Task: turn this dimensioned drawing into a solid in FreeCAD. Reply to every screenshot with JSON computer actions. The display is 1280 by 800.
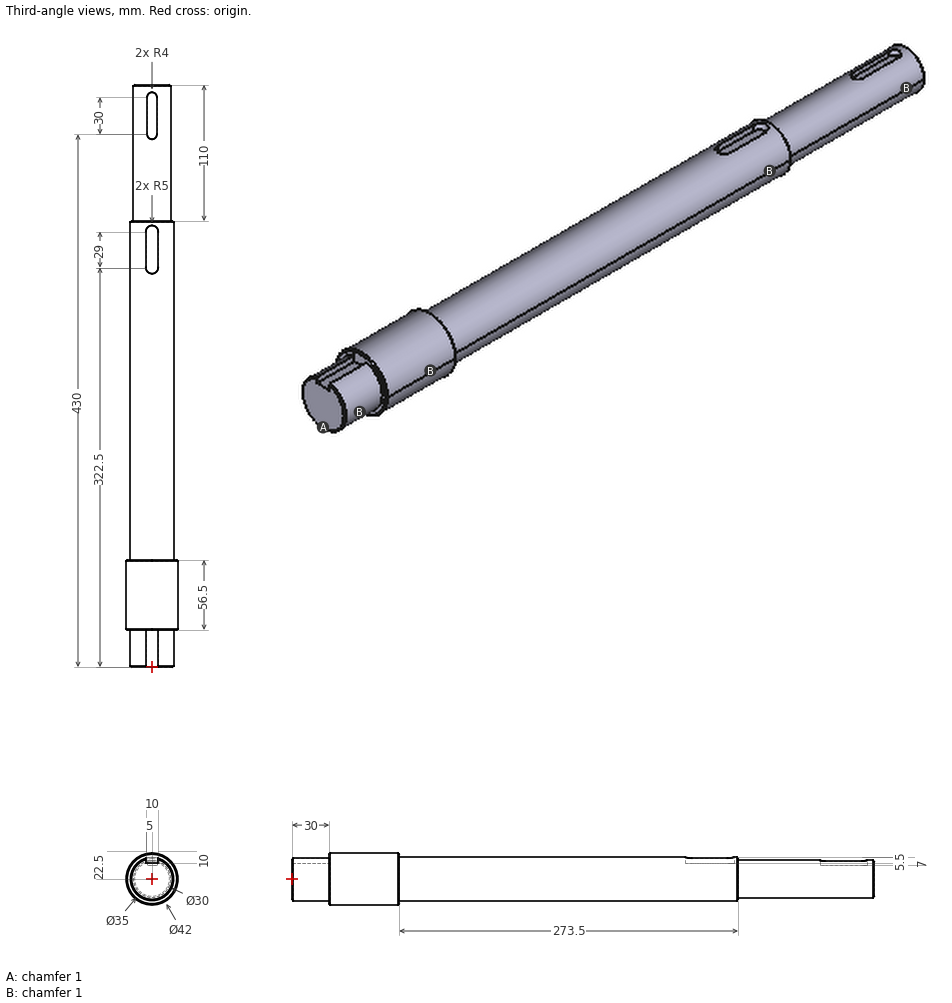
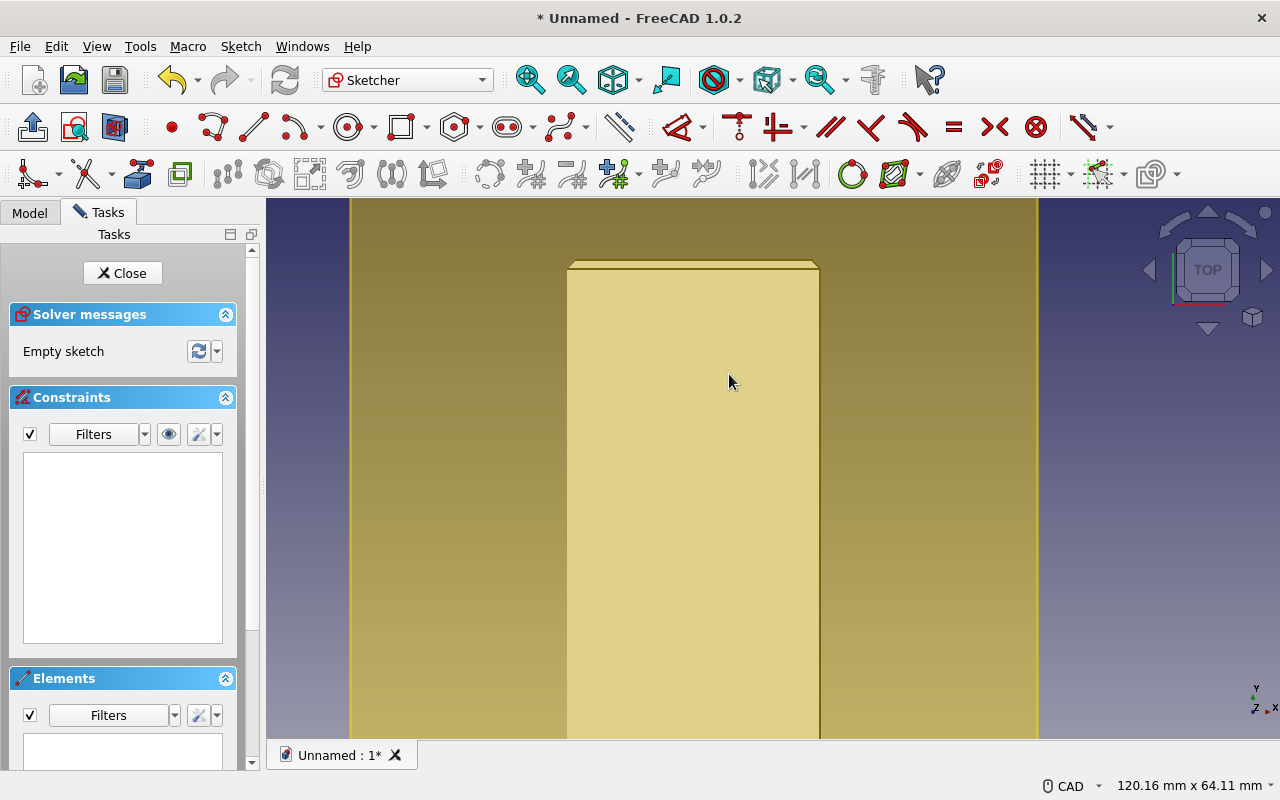
{"action": "key", "text": "g s"}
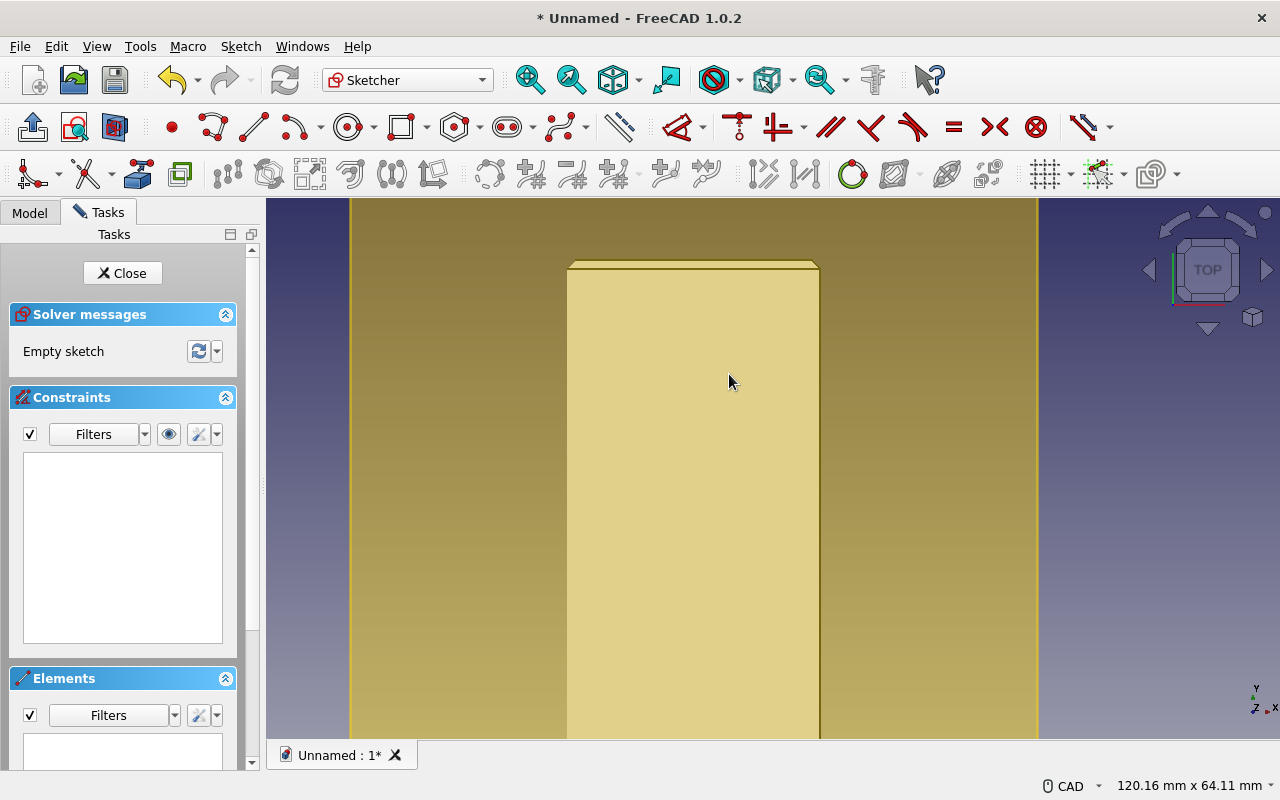
{"action": "left_click", "coordinate": [694, 598]}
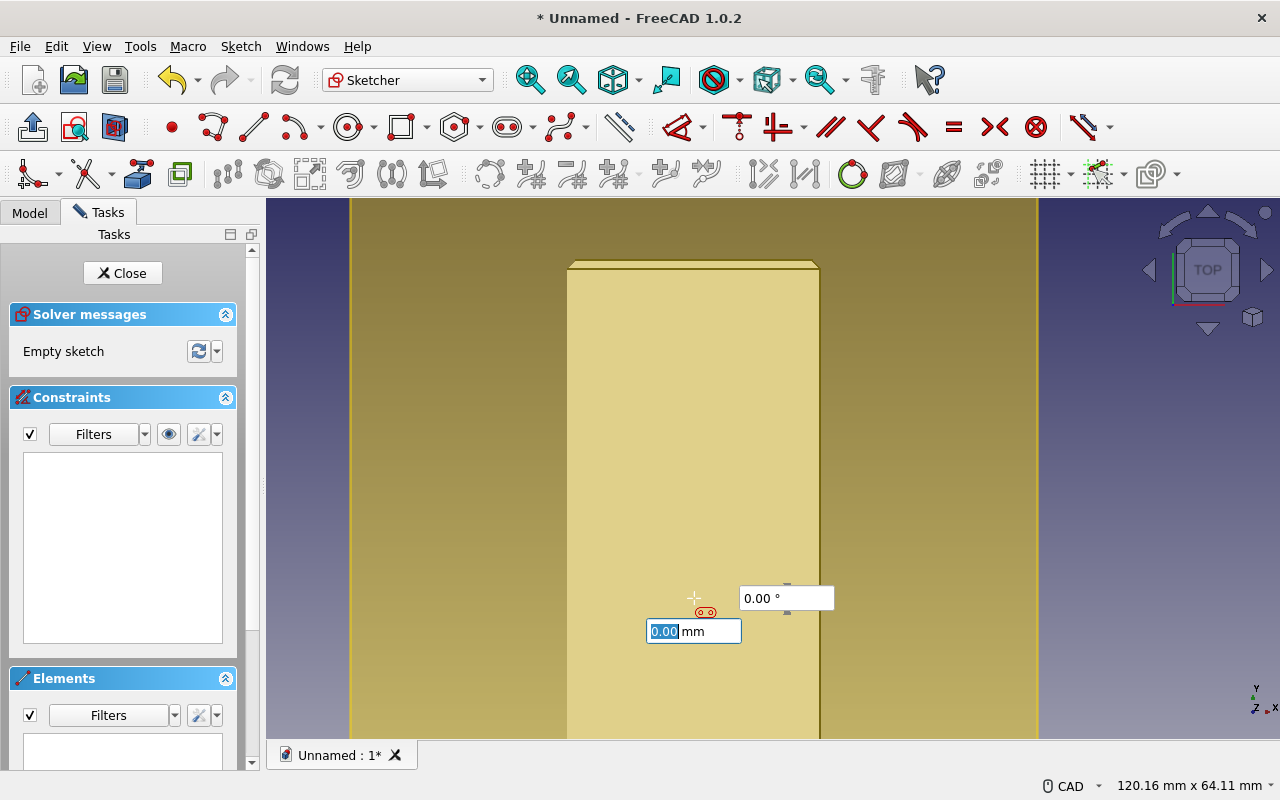
{"action": "left_click", "coordinate": [703, 345]}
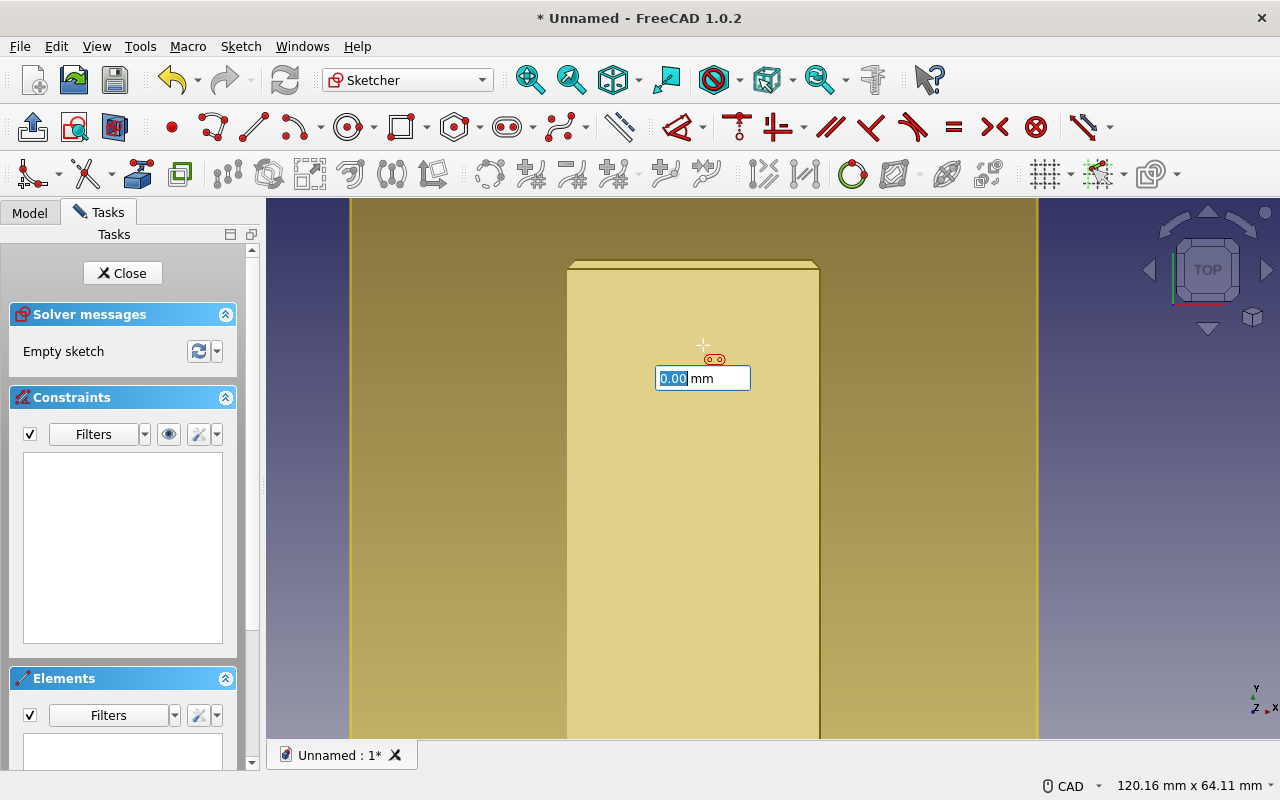
{"action": "left_click", "coordinate": [728, 471]}
{"action": "key", "text": "Escape"}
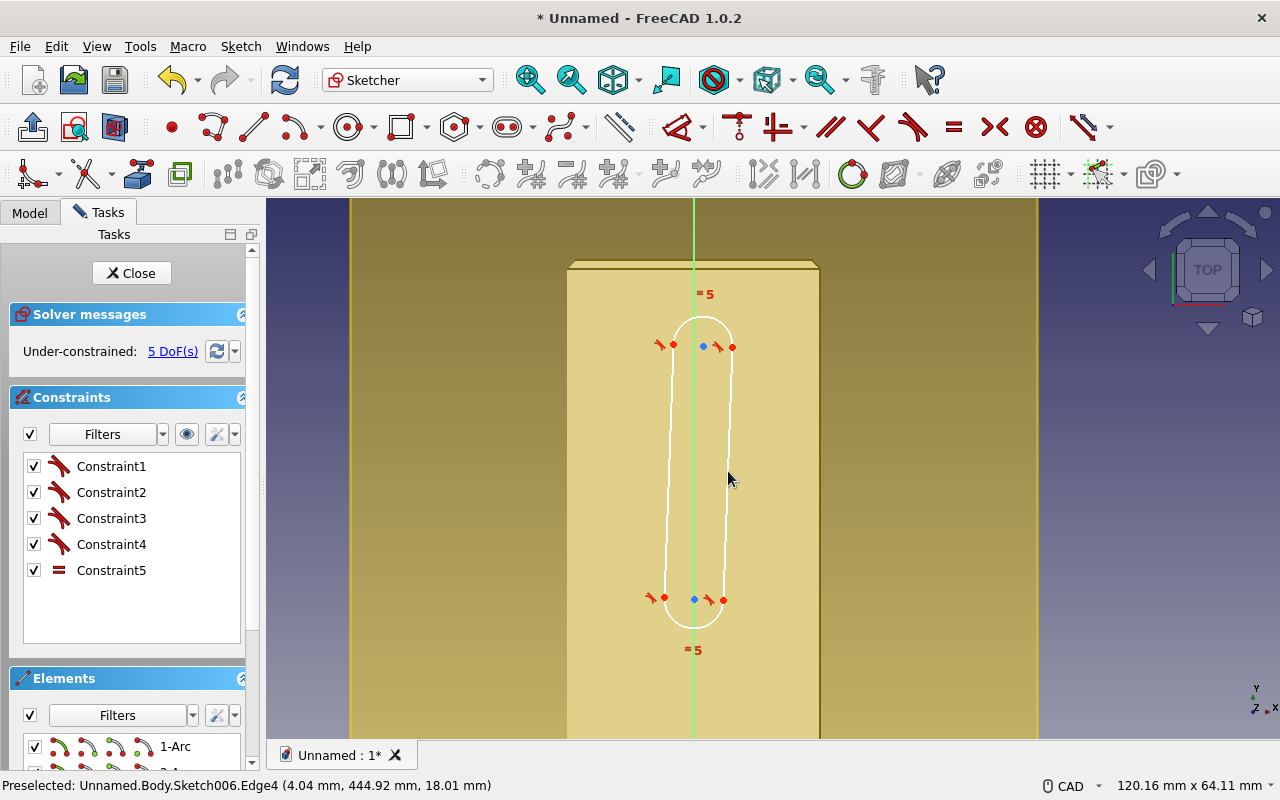
{"action": "left_click", "coordinate": [667, 522]}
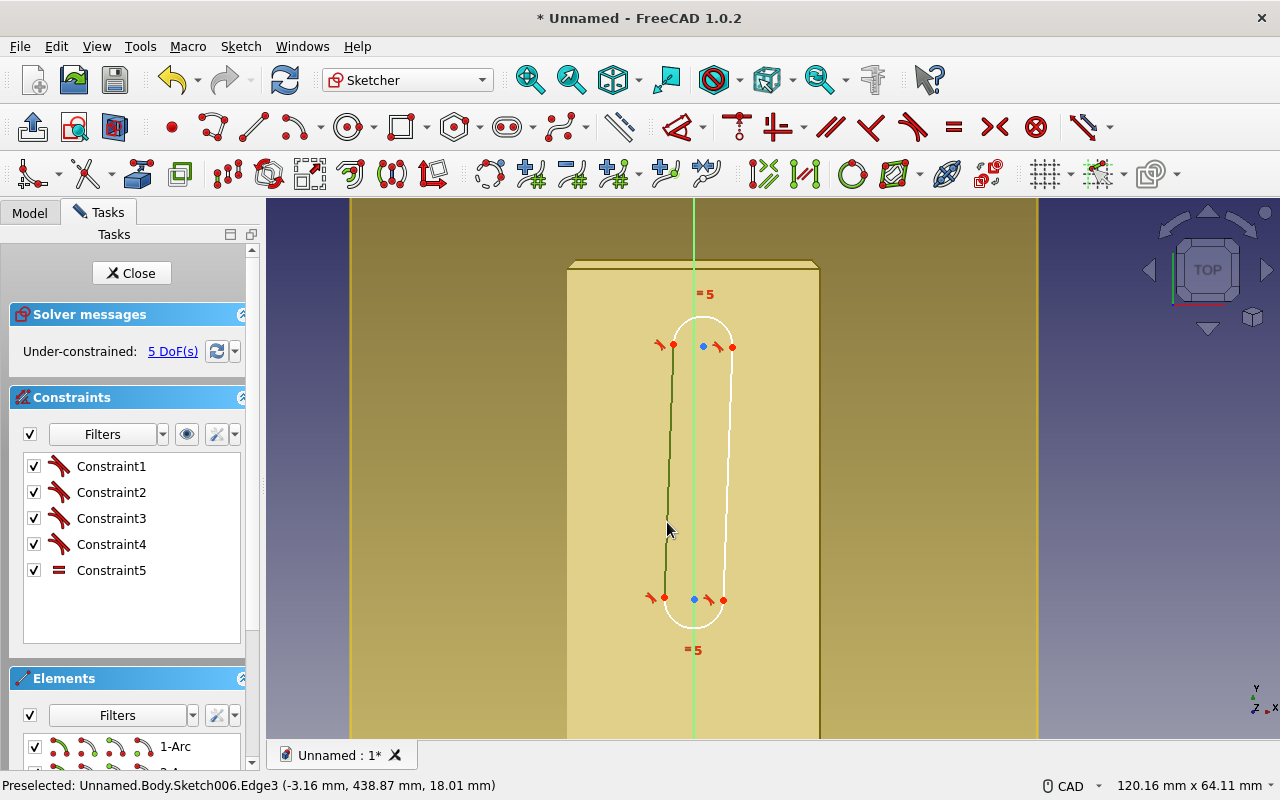
{"action": "key", "text": "v"}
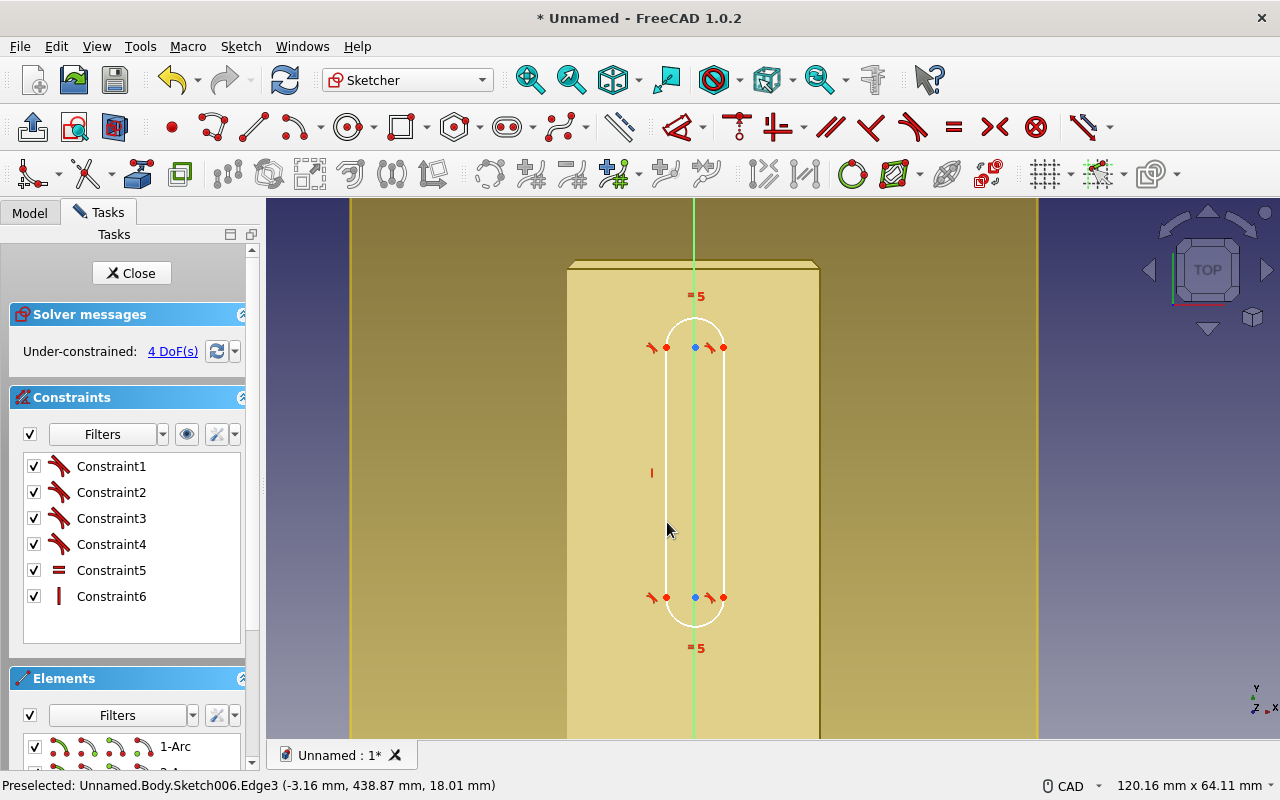
{"action": "left_click", "coordinate": [695, 598]}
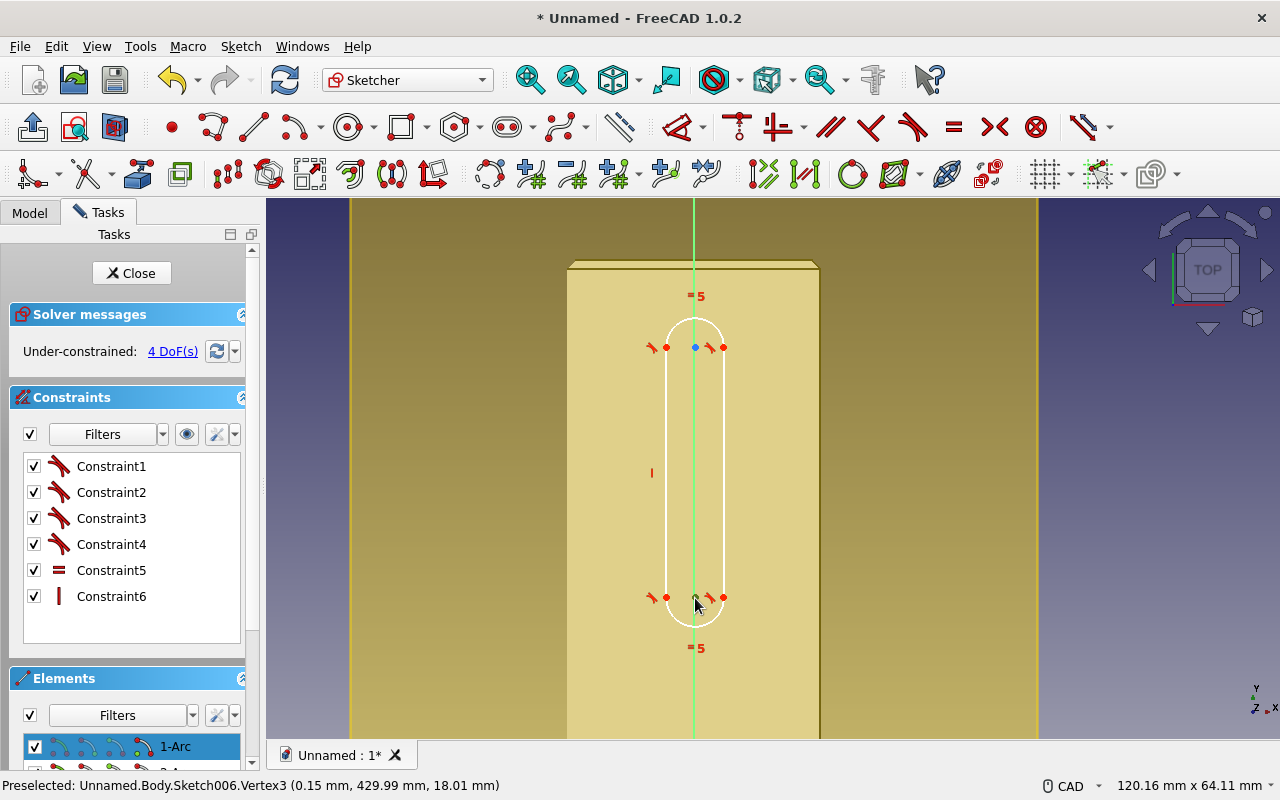
{"action": "left_click", "coordinate": [694, 676]}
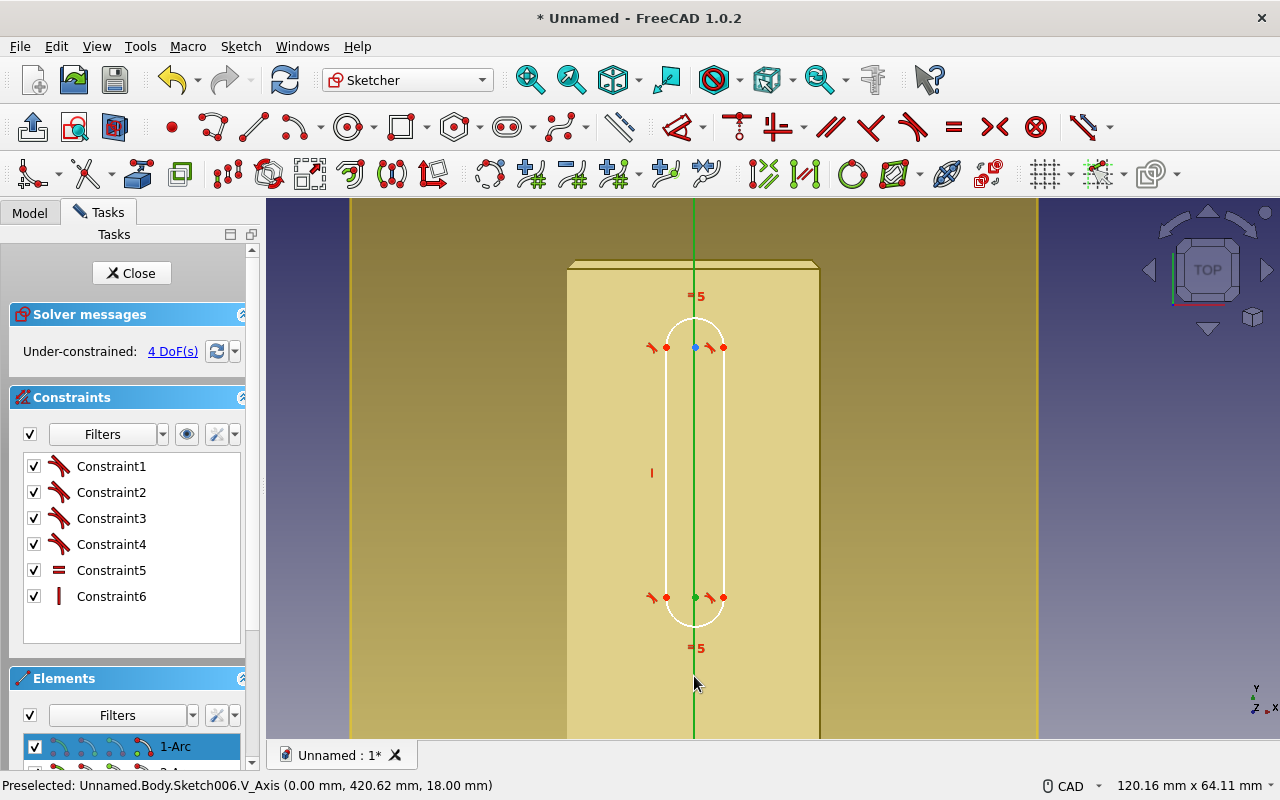
{"action": "key", "text": "c"}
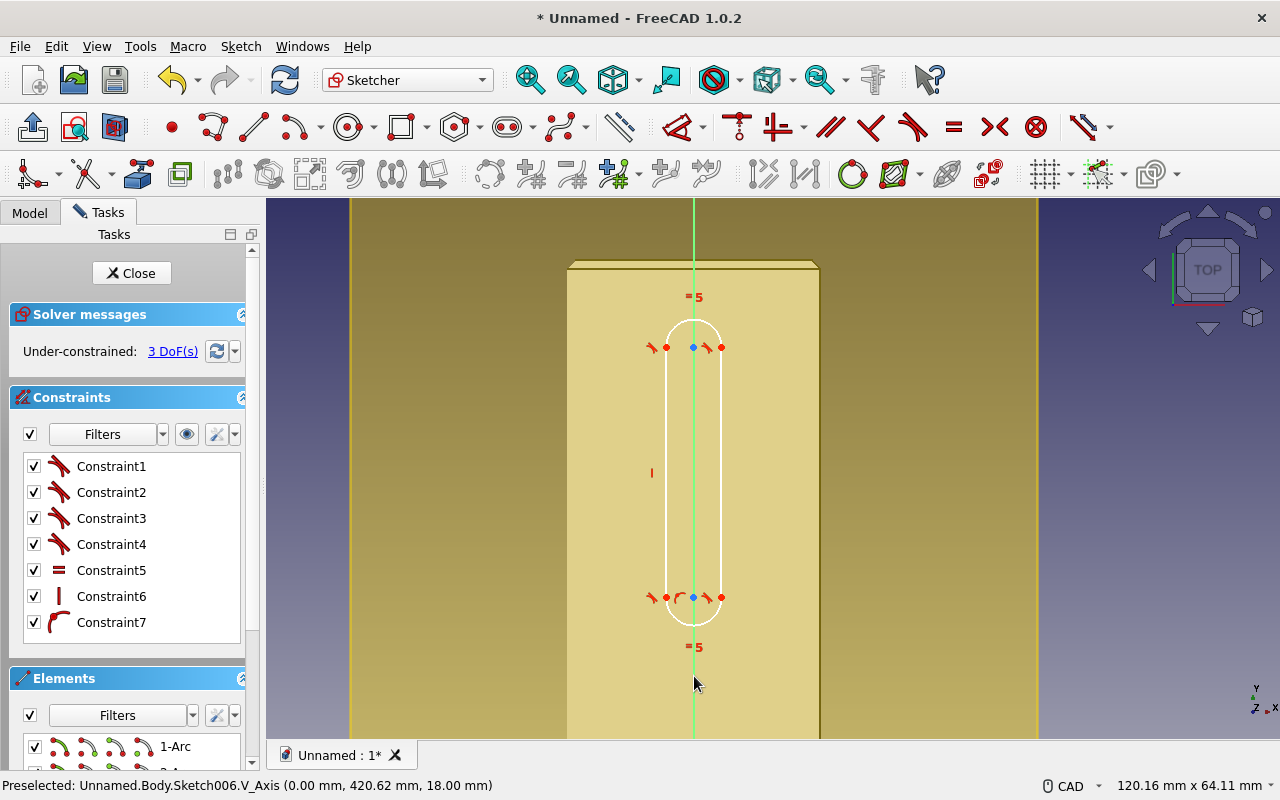
{"action": "key", "text": "d"}